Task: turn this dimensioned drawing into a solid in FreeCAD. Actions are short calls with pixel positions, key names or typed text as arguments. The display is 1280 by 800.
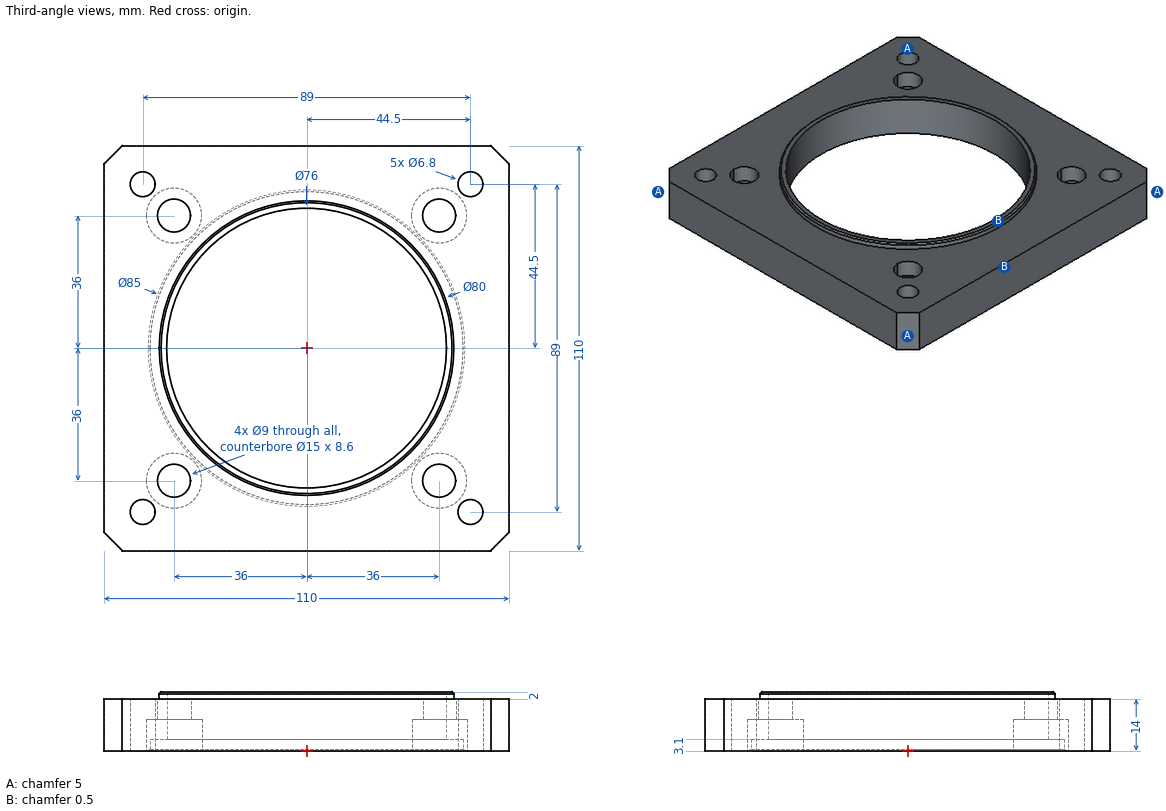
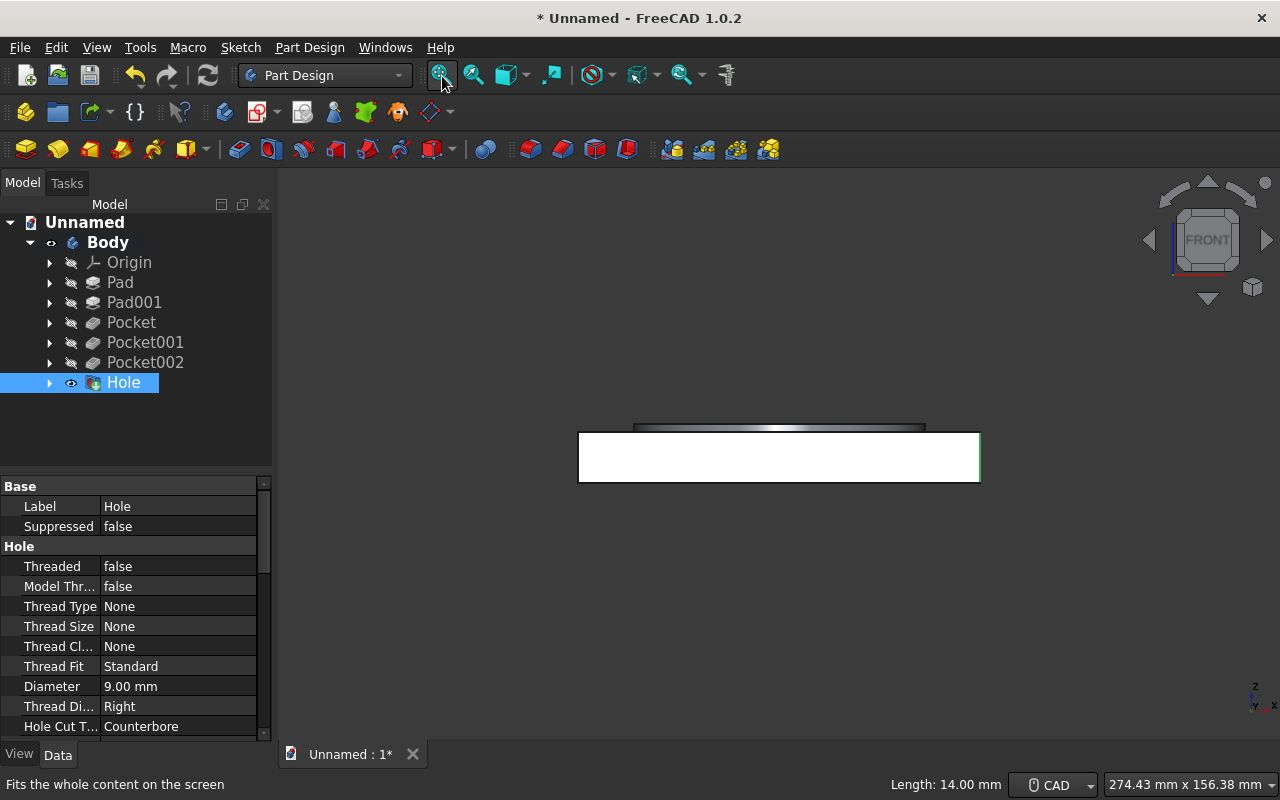
click(578, 456, ctrl)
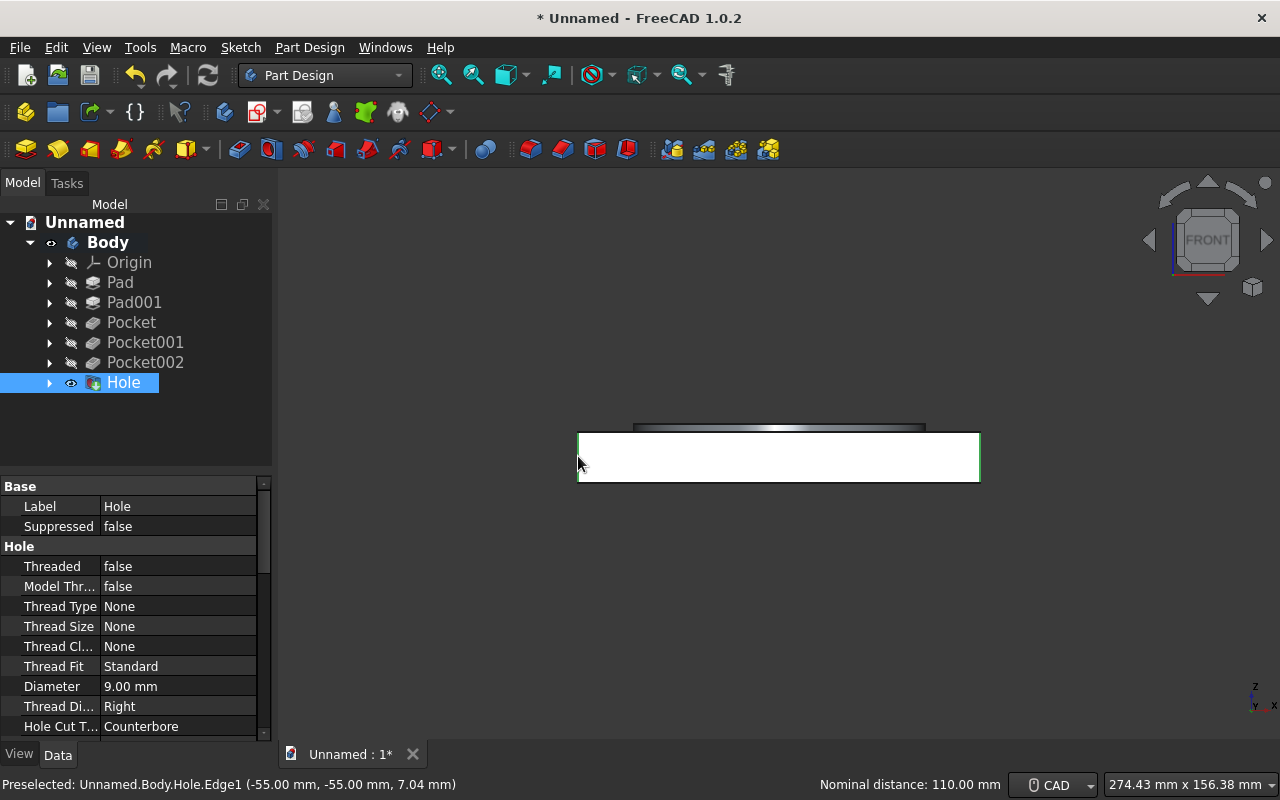
key(3)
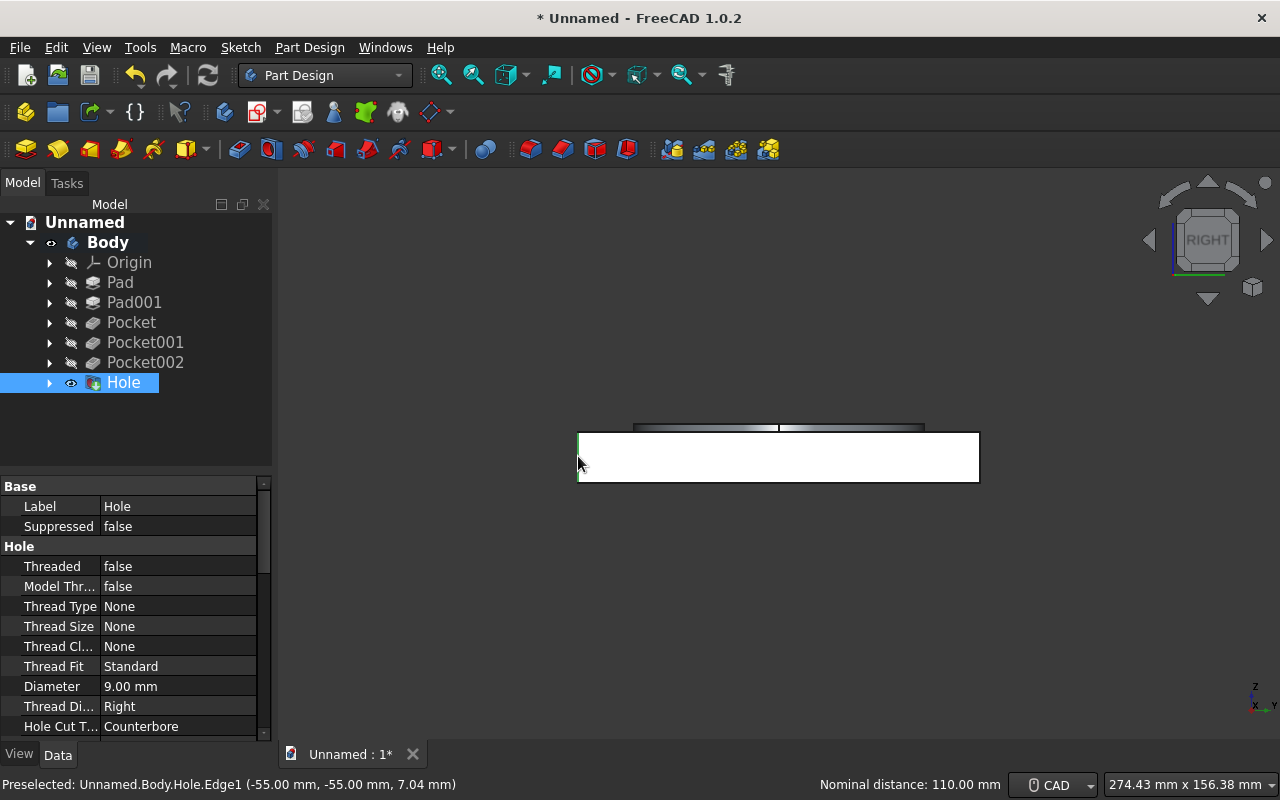
click(442, 76)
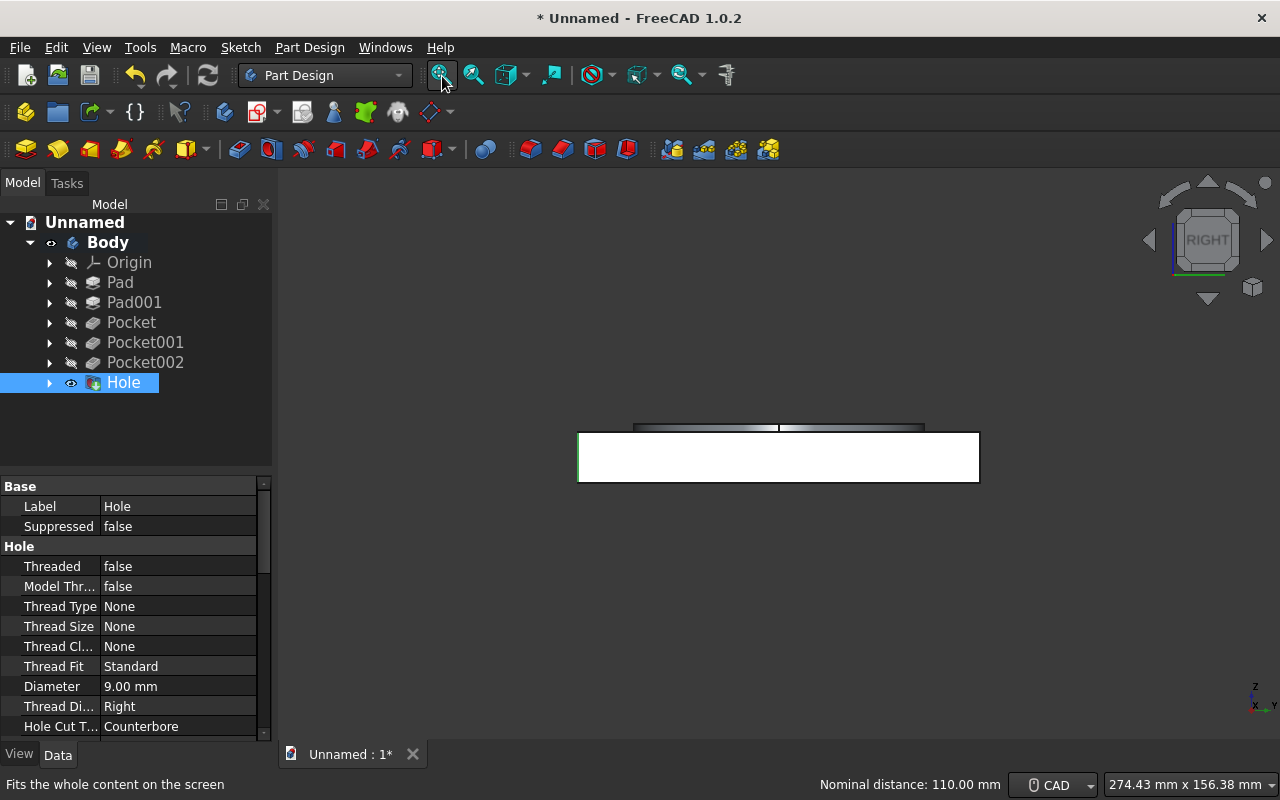
click(980, 456, ctrl)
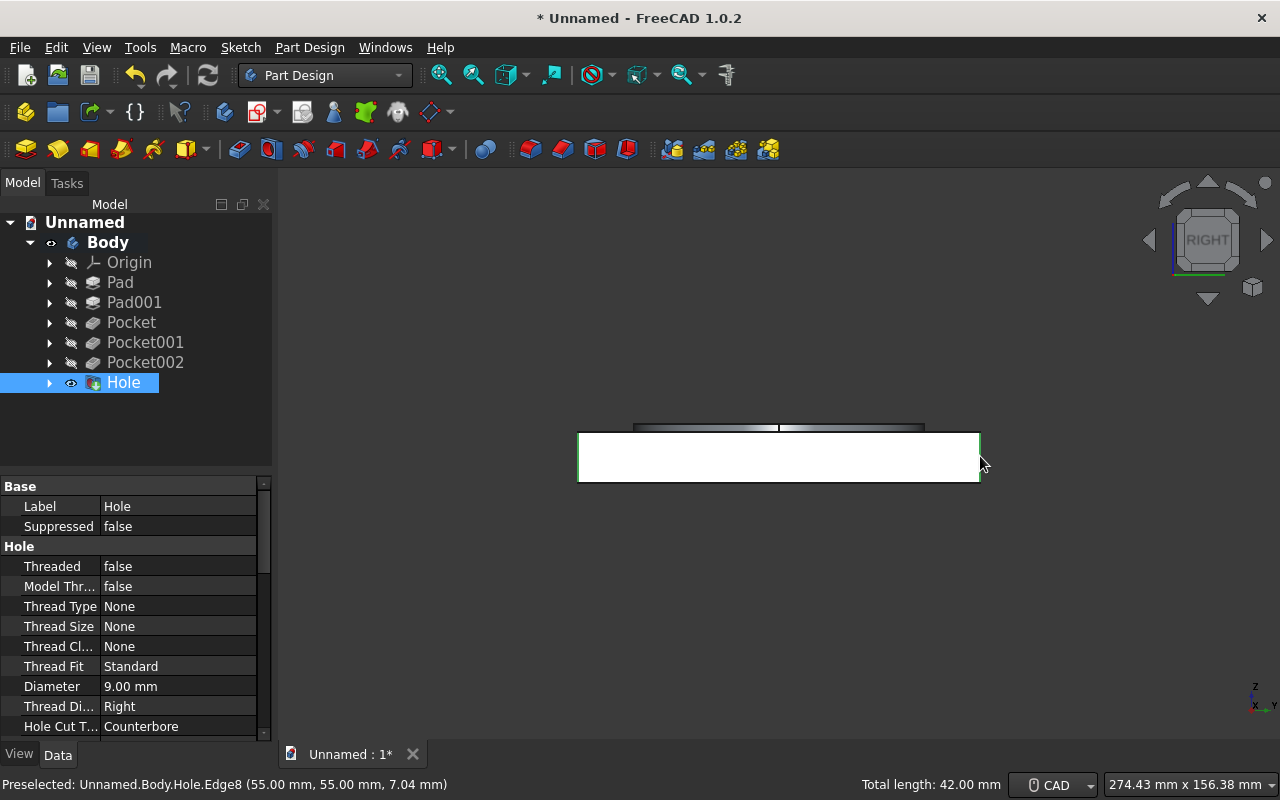
key(5)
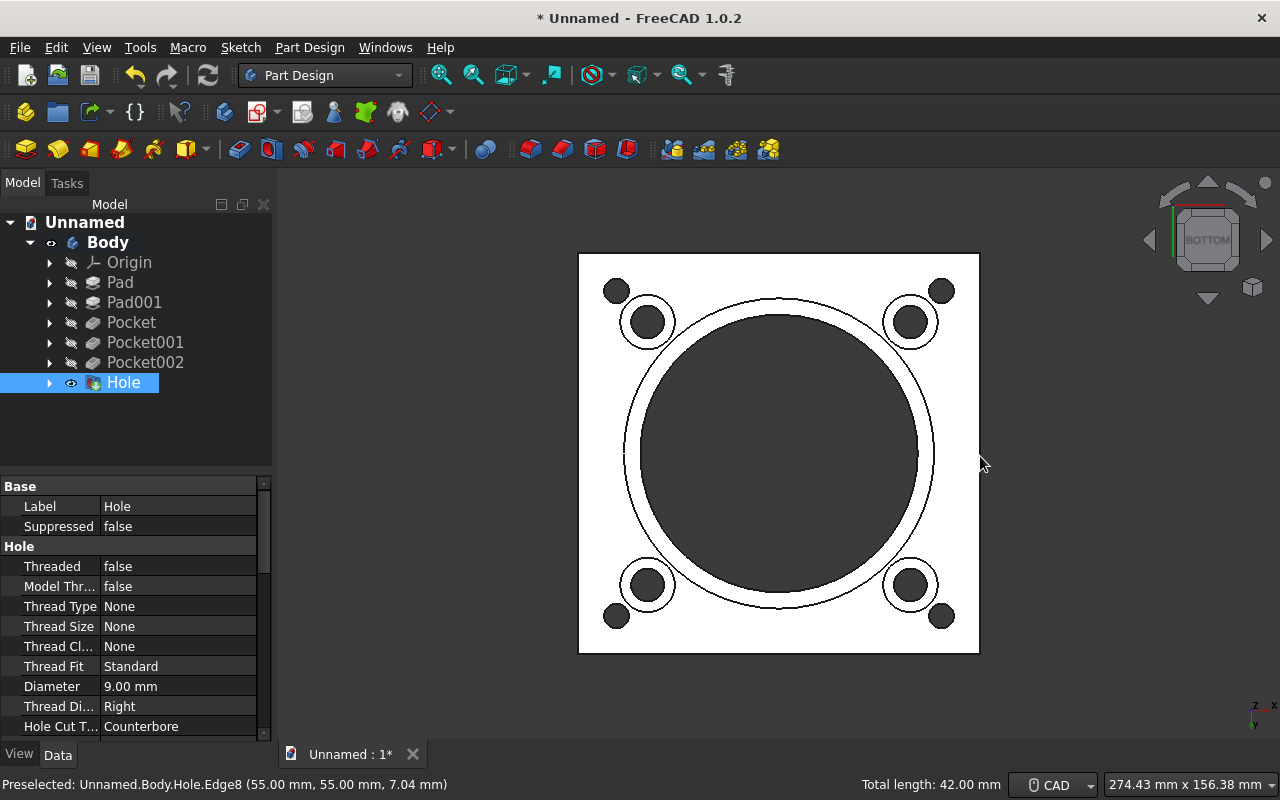
key(4)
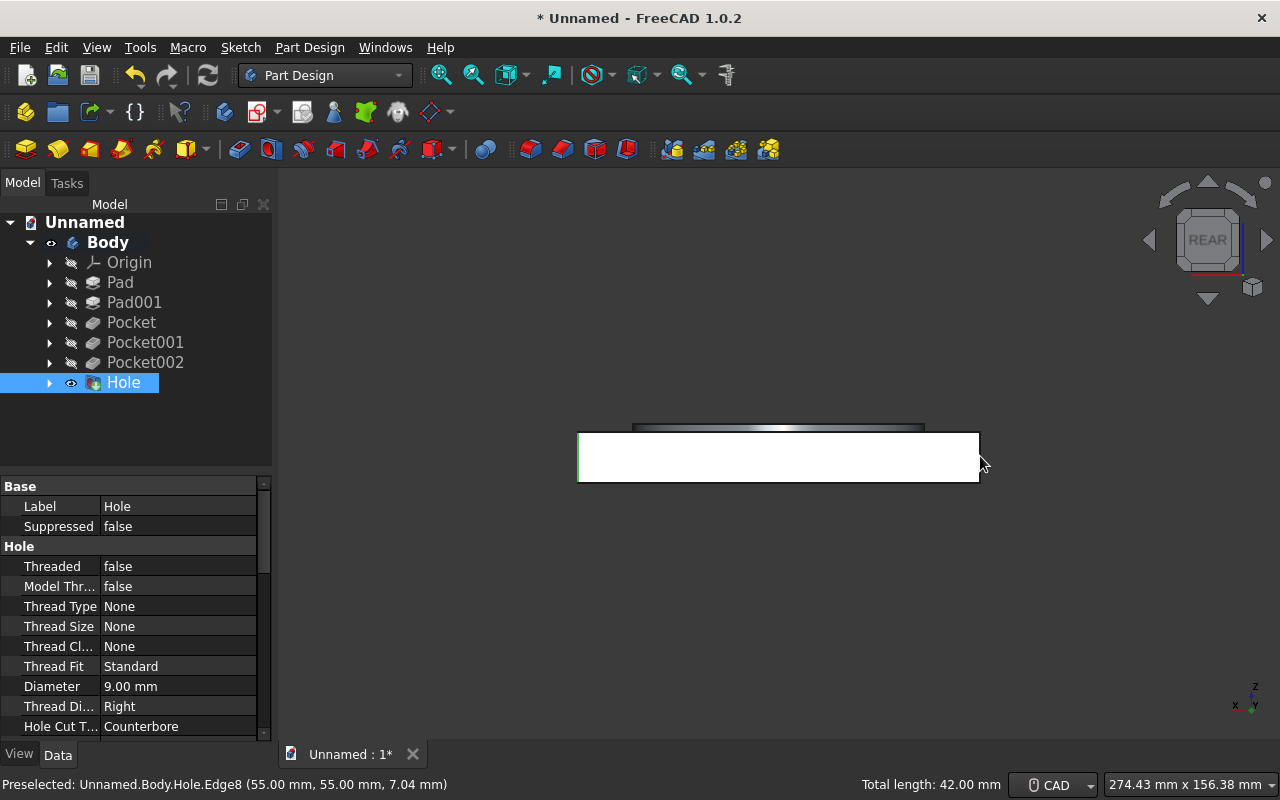
click(442, 76)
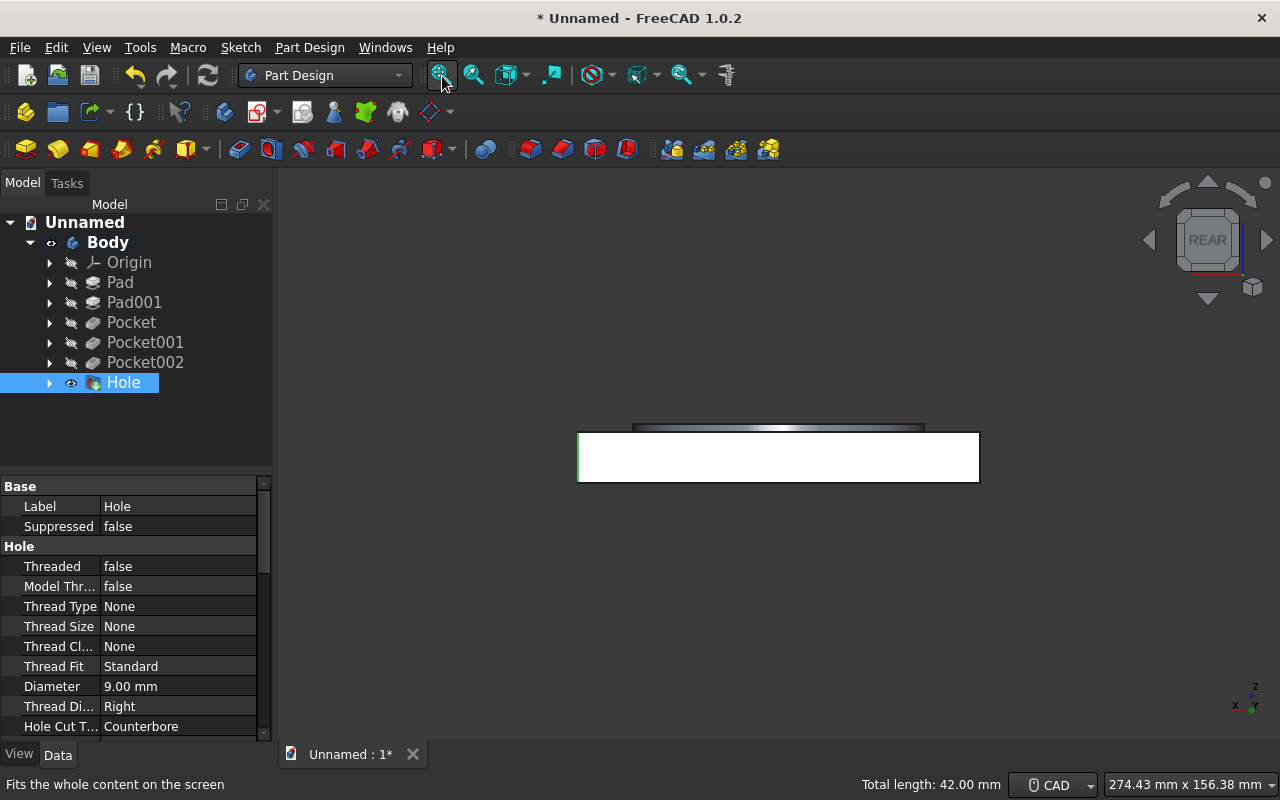
click(980, 456, ctrl)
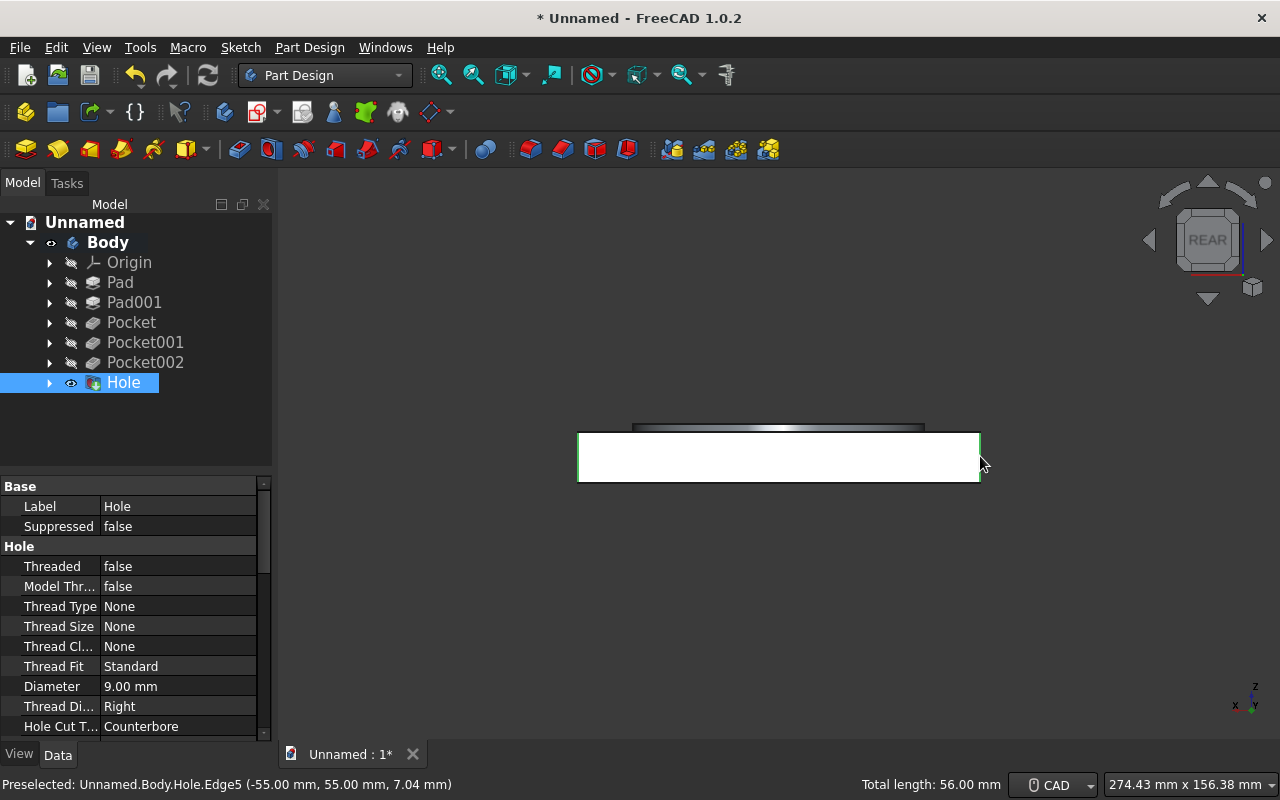
click(564, 150)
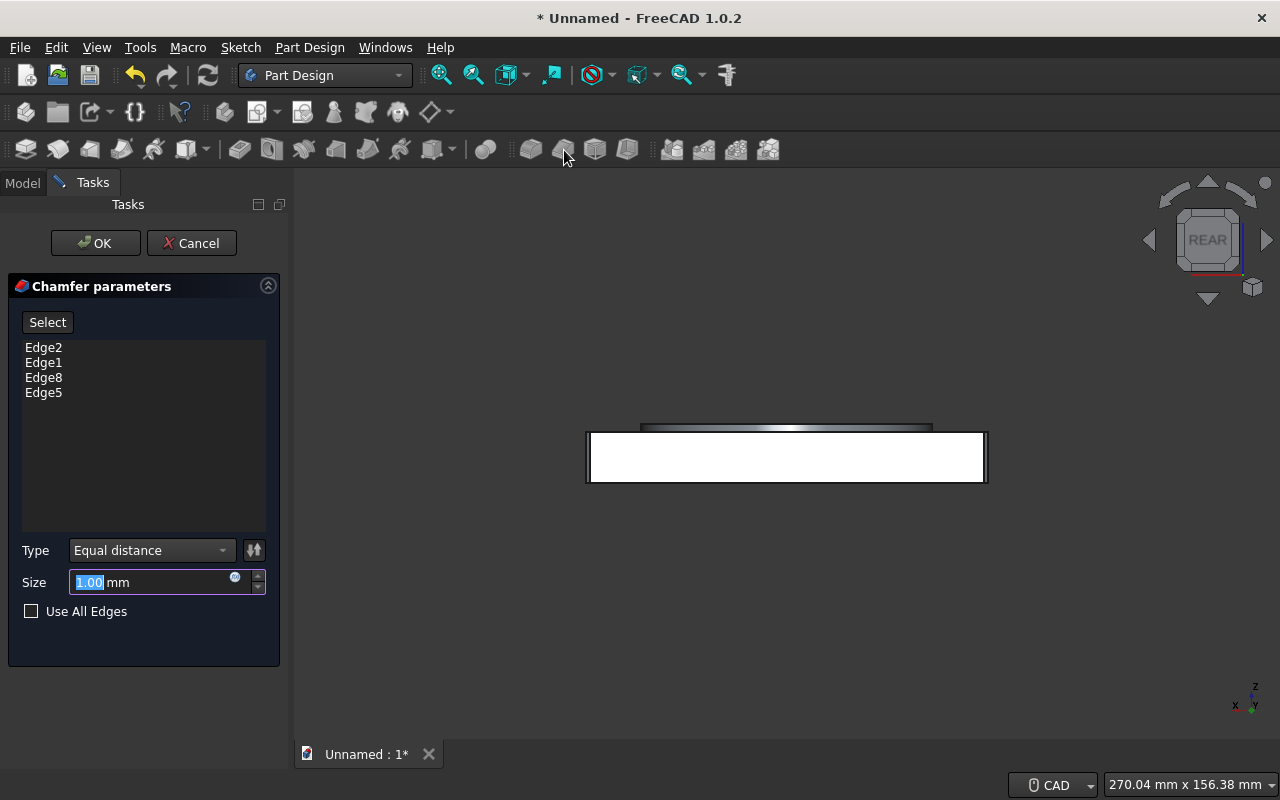
text(5)
key(Tab)